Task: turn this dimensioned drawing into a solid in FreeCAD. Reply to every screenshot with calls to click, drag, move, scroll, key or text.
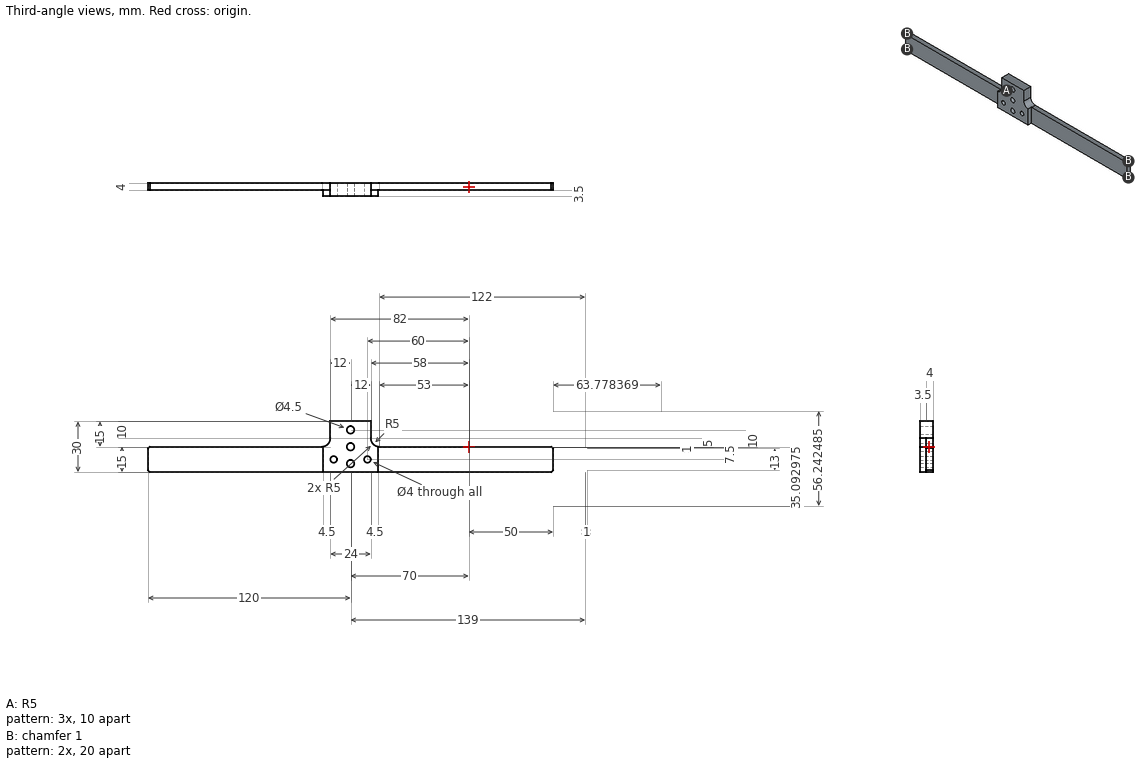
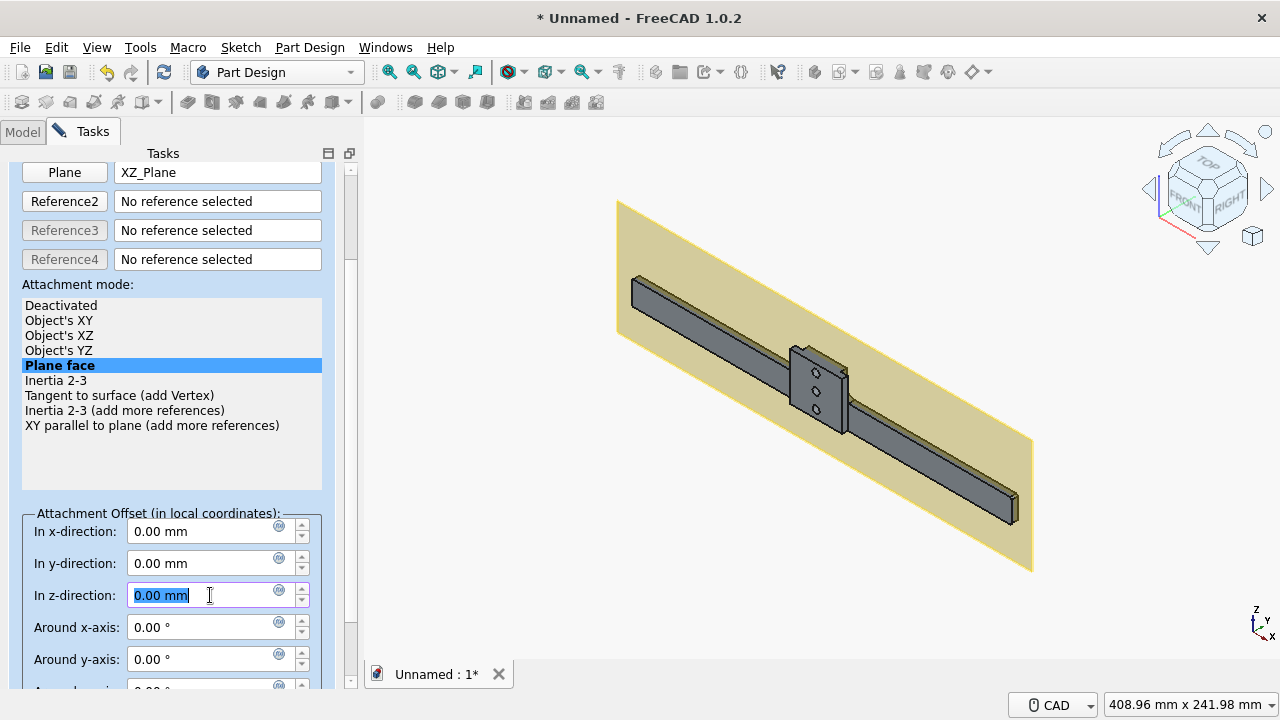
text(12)
key(Tab)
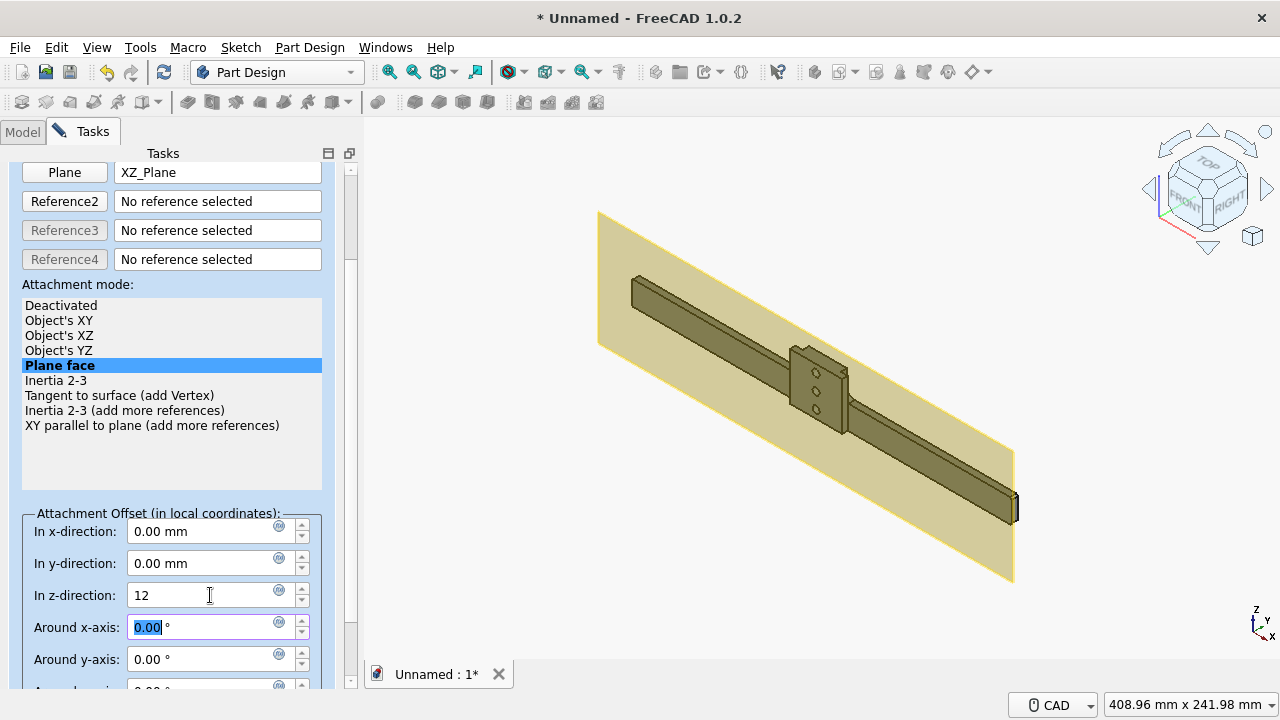
scroll(351, 426, up, 3)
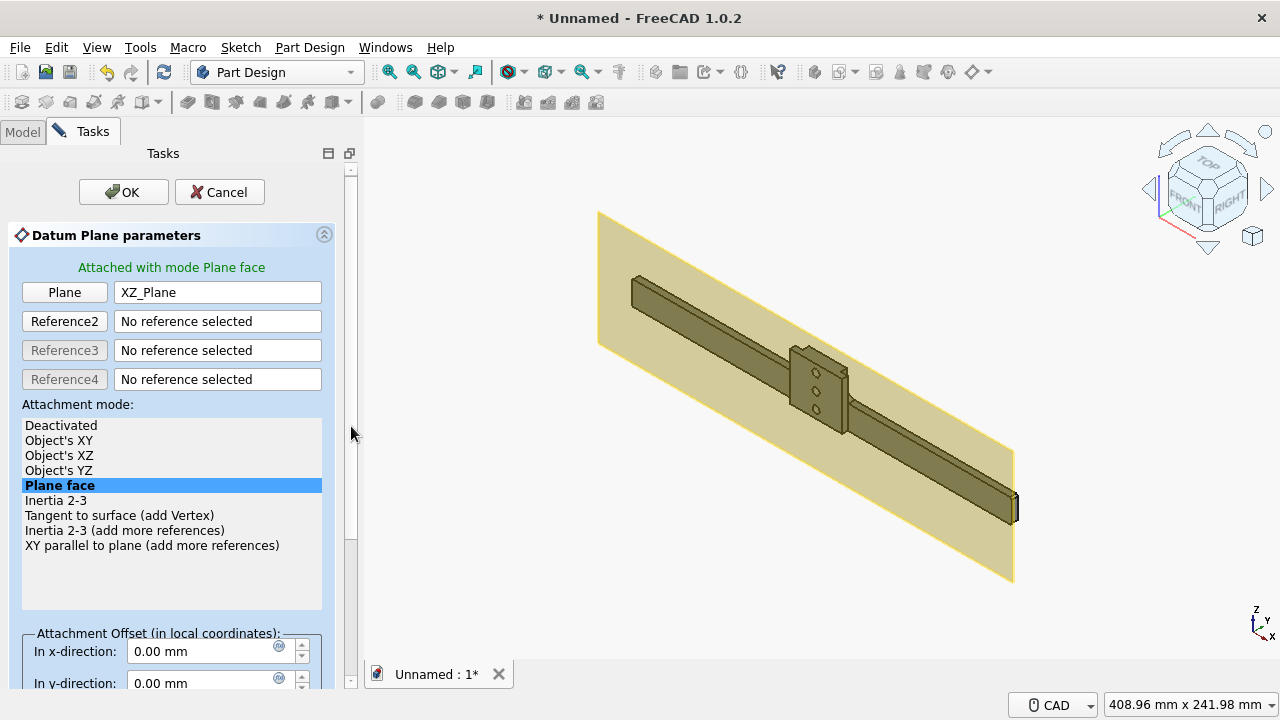
click(124, 192)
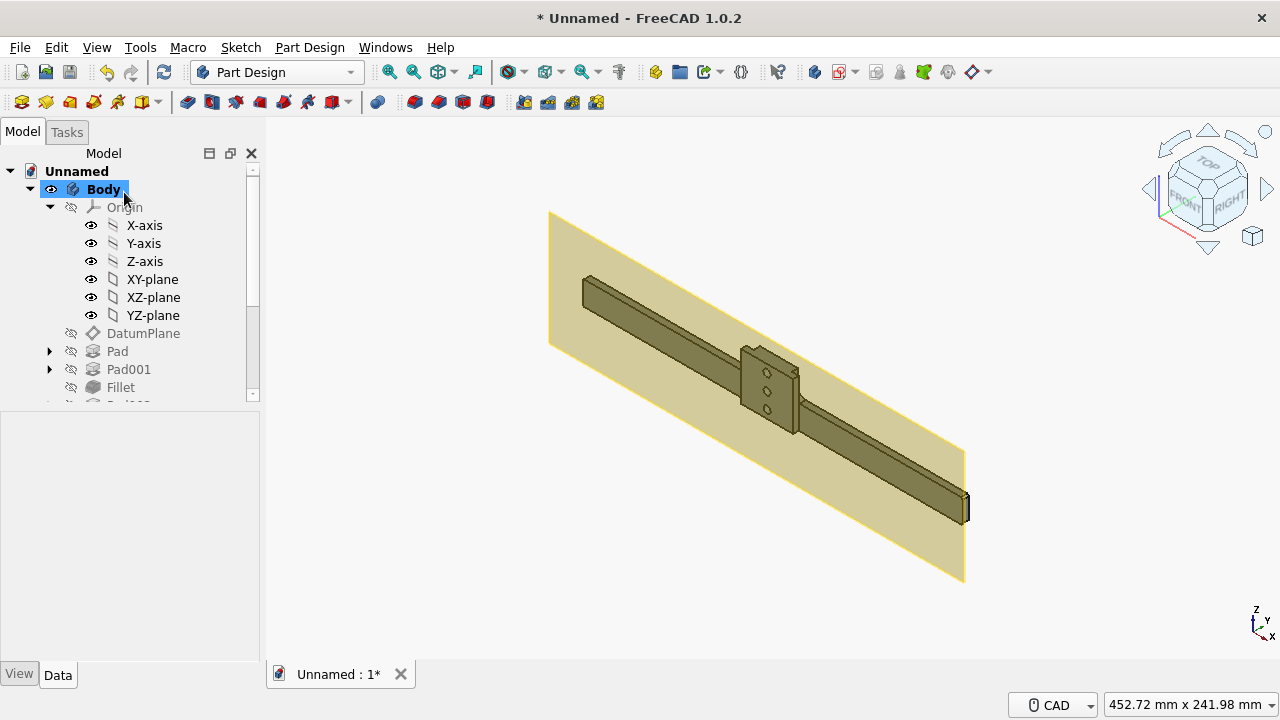
scroll(100, 275, down, 3)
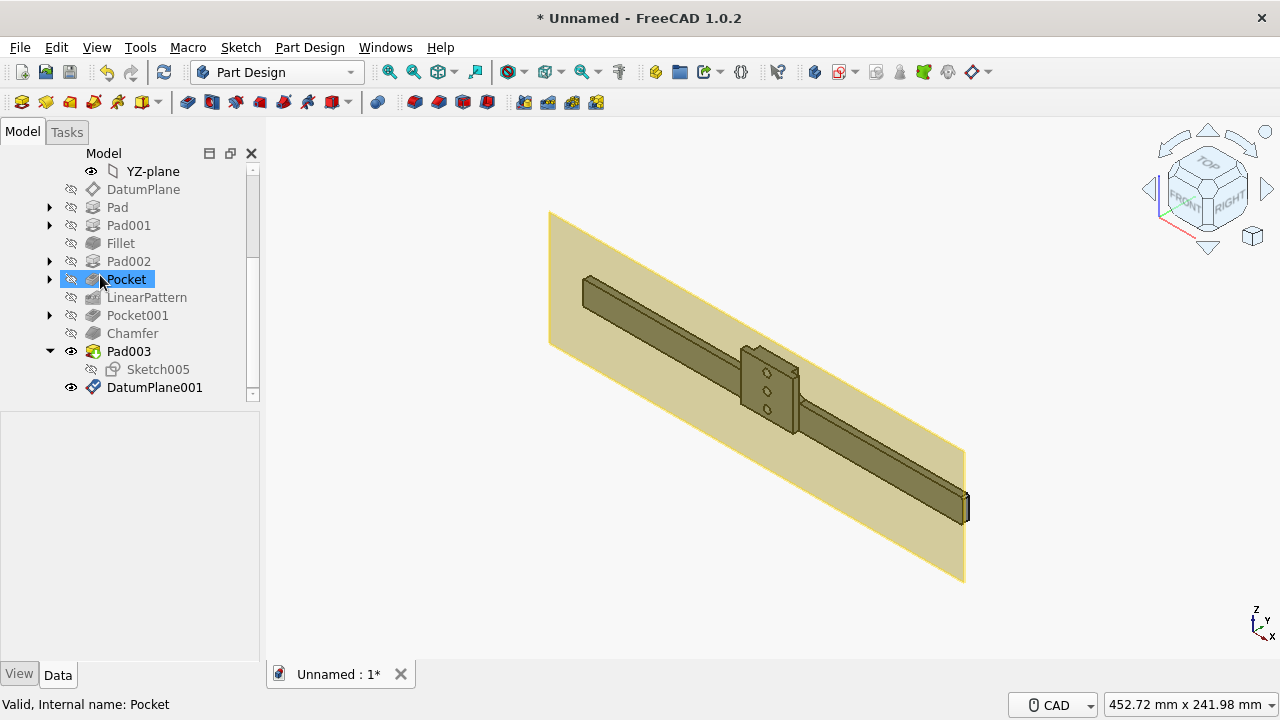
click(116, 387)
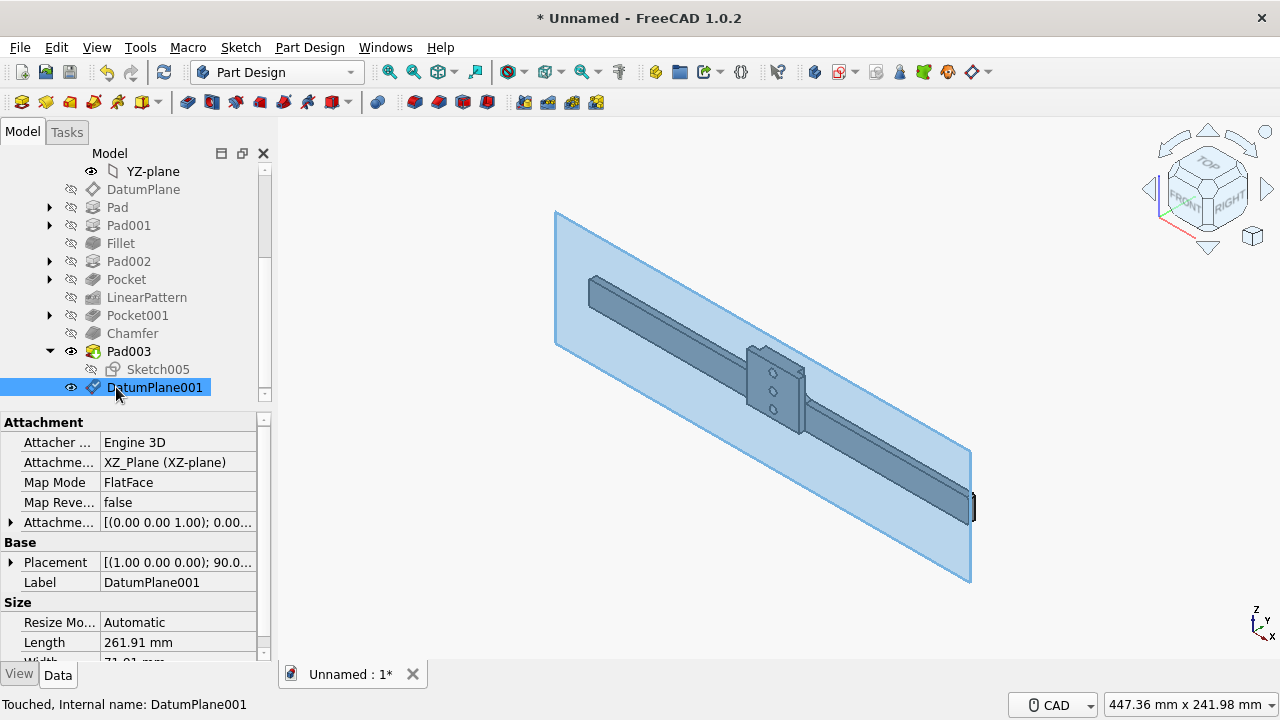
click(840, 72)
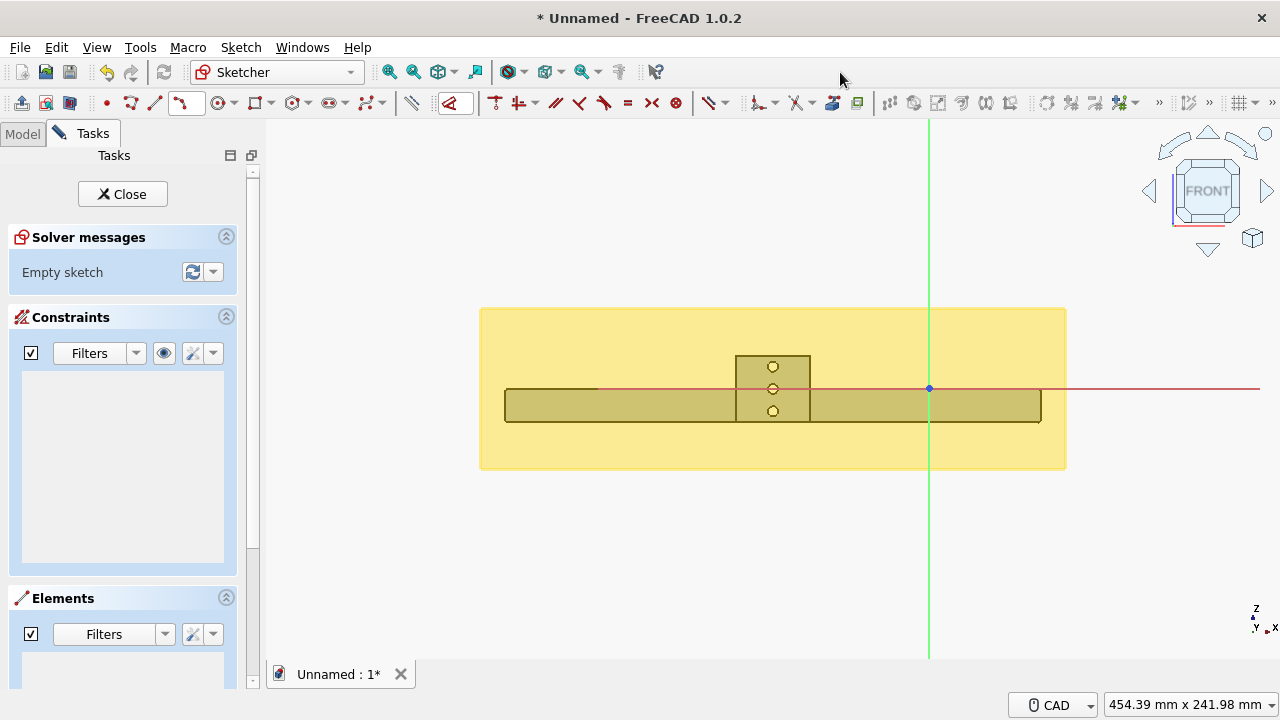
scroll(784, 370, up, 10)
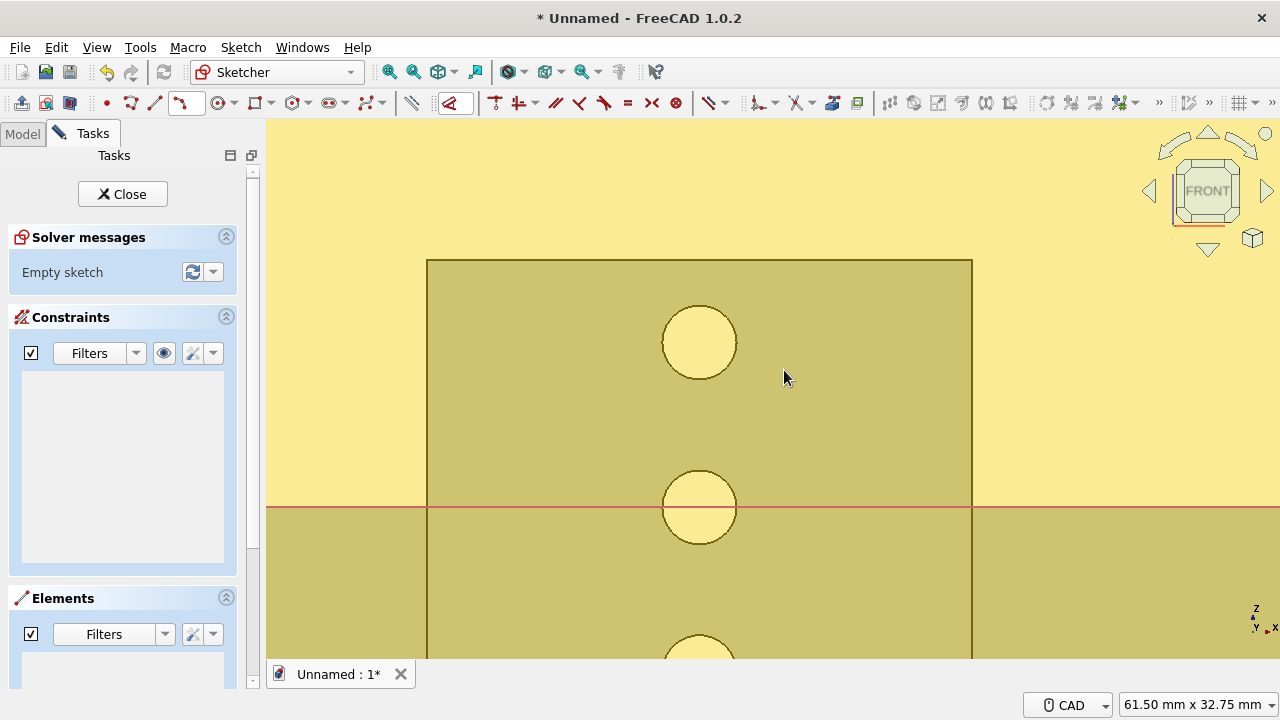
click(132, 104)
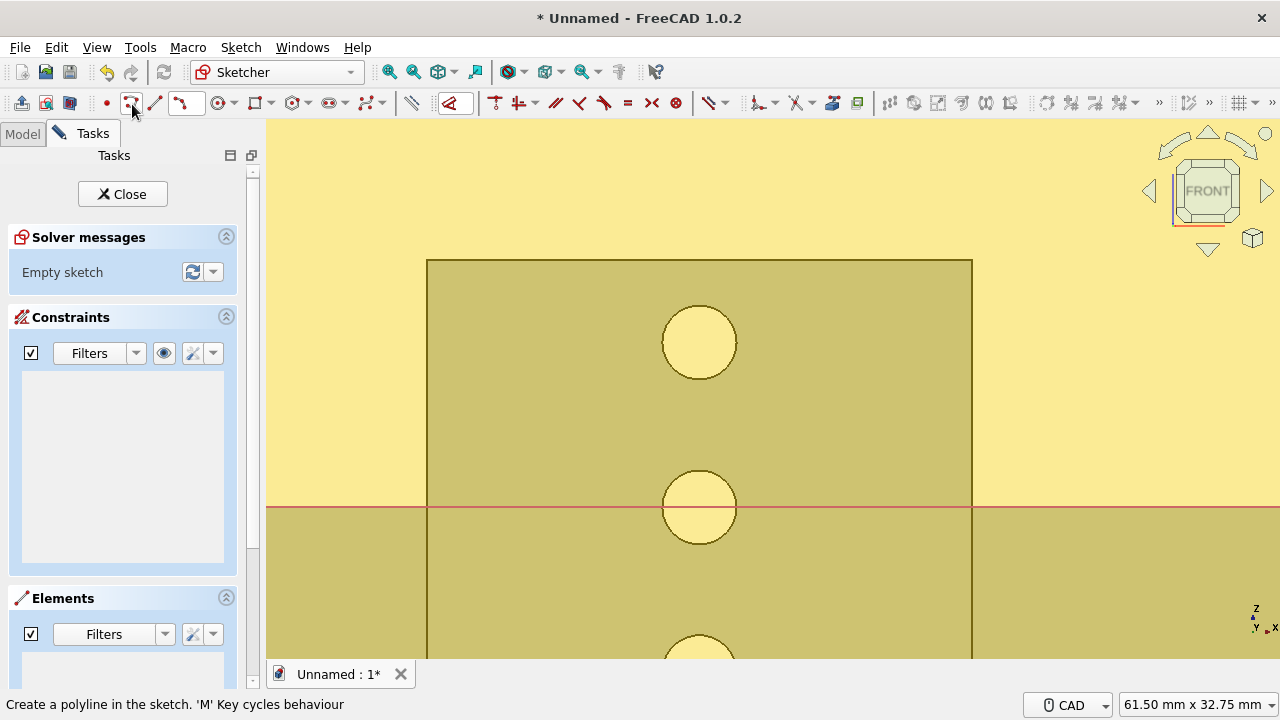
click(897, 425)
click(897, 260)
click(972, 260)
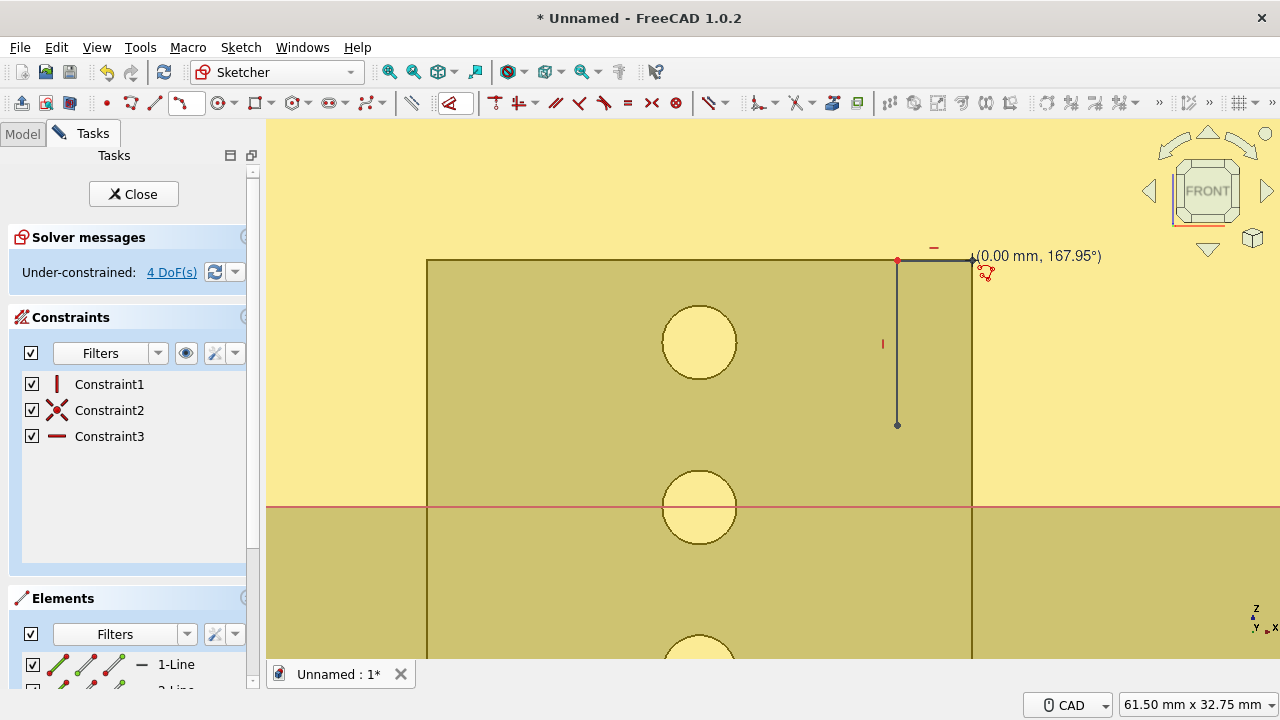
scroll(972, 507, up, 19)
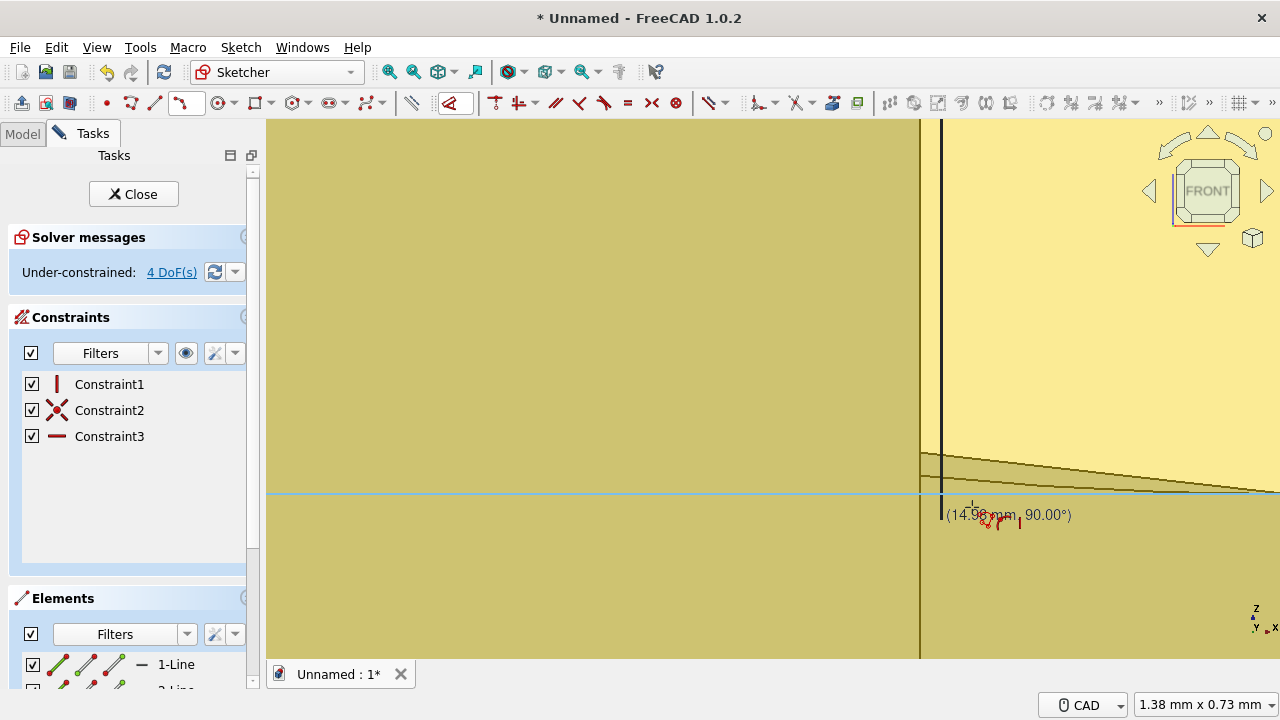
click(942, 476)
right_click(942, 476)